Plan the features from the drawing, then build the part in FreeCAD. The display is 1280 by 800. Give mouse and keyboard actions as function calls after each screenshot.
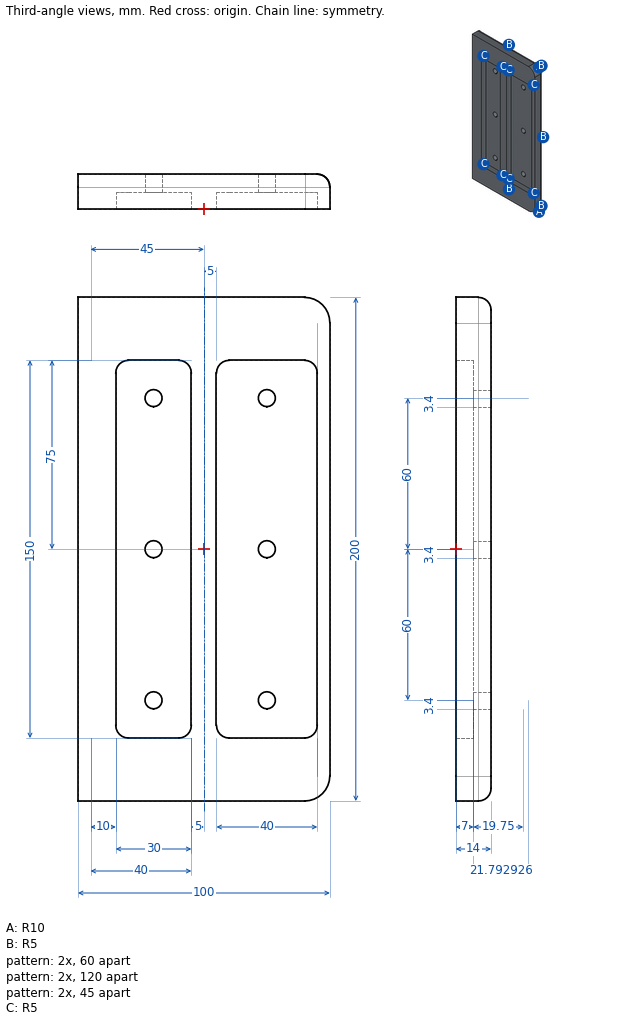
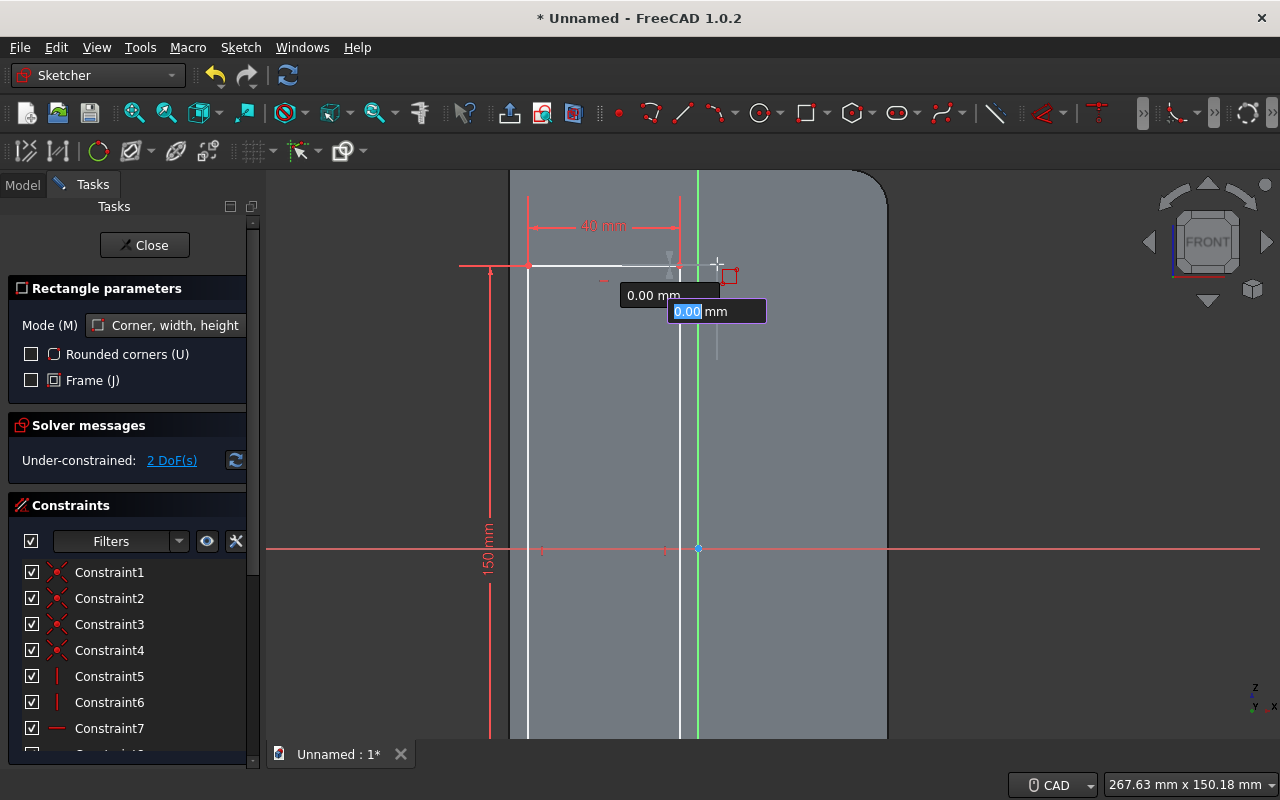
scroll(717, 263, down, 2)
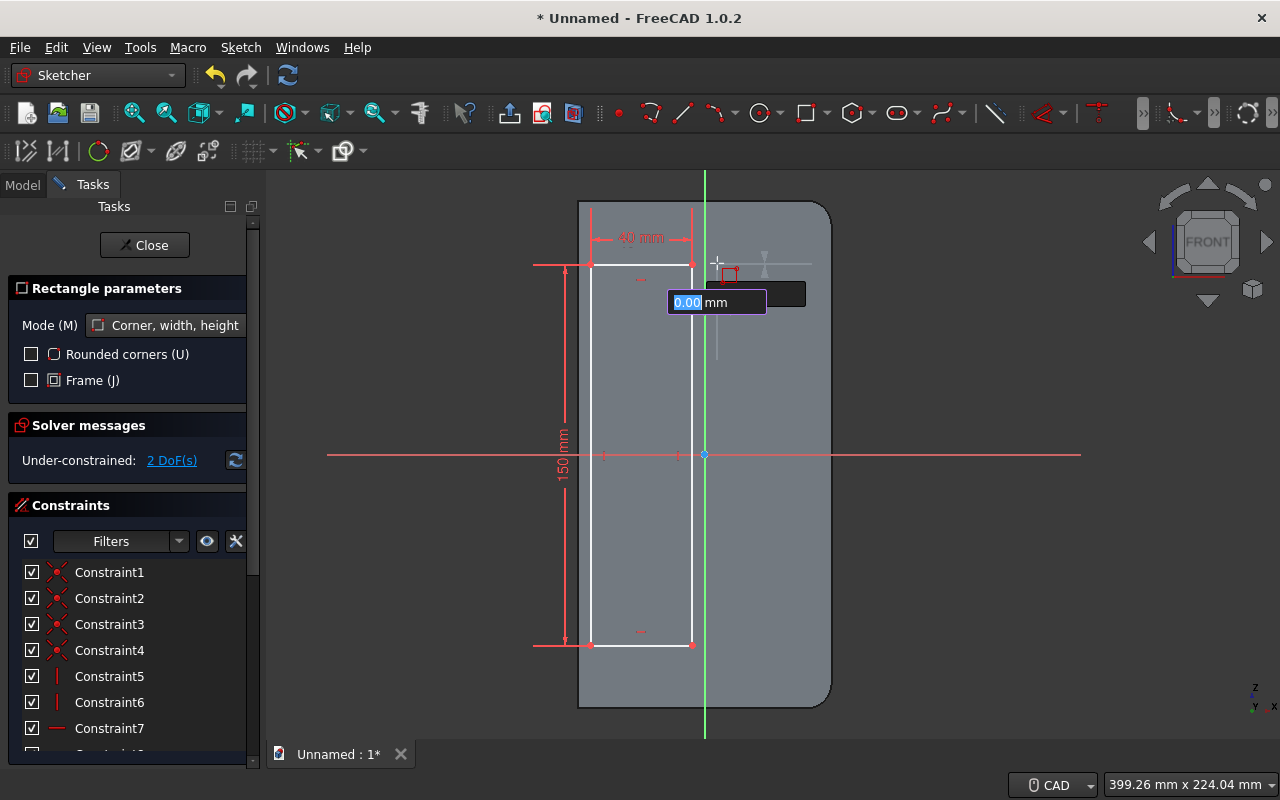
click(819, 645)
key(Escape)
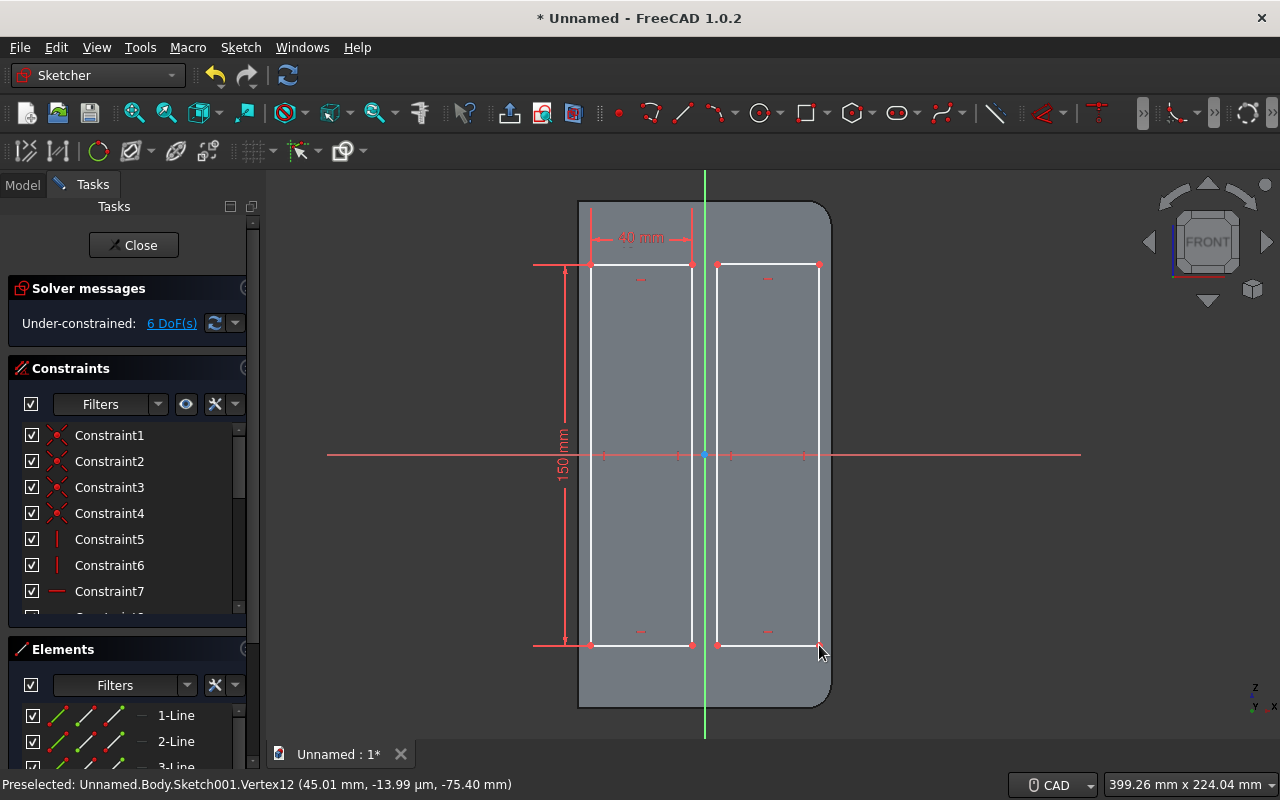
click(692, 265)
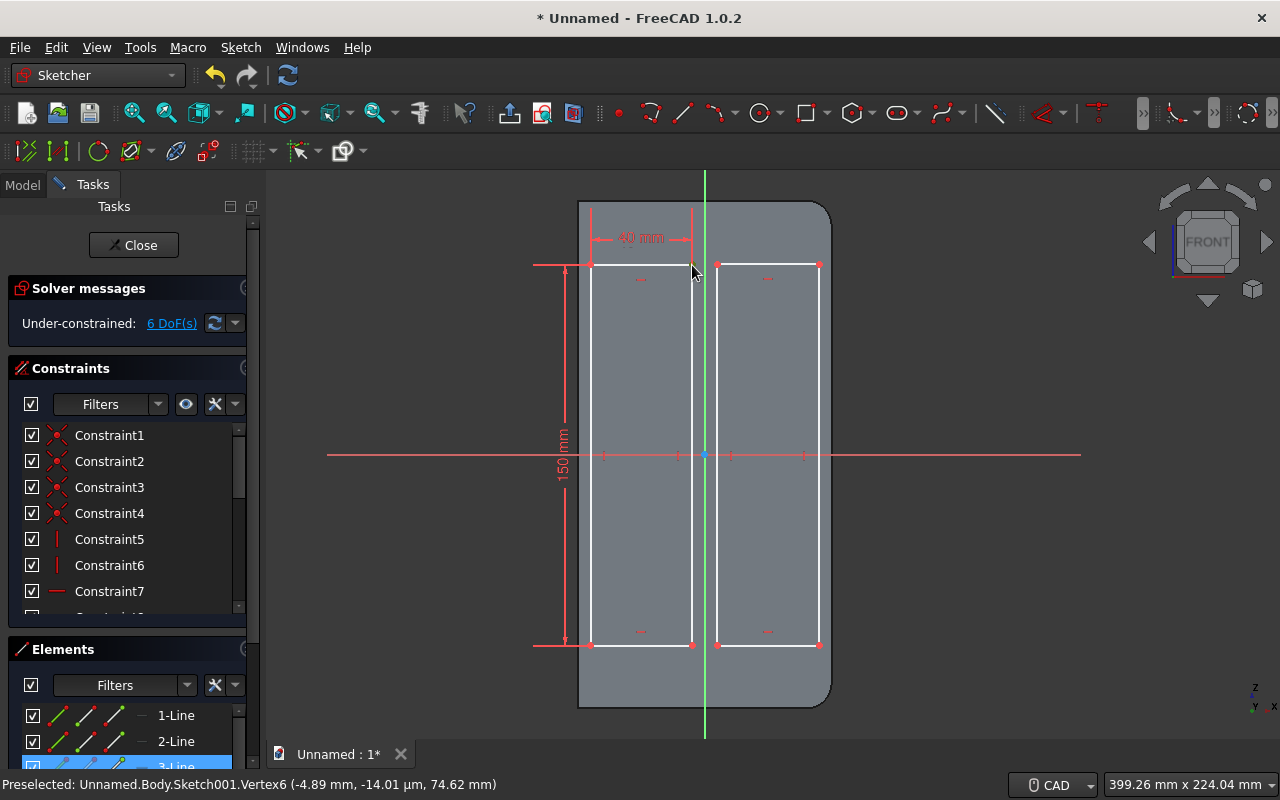
click(717, 264)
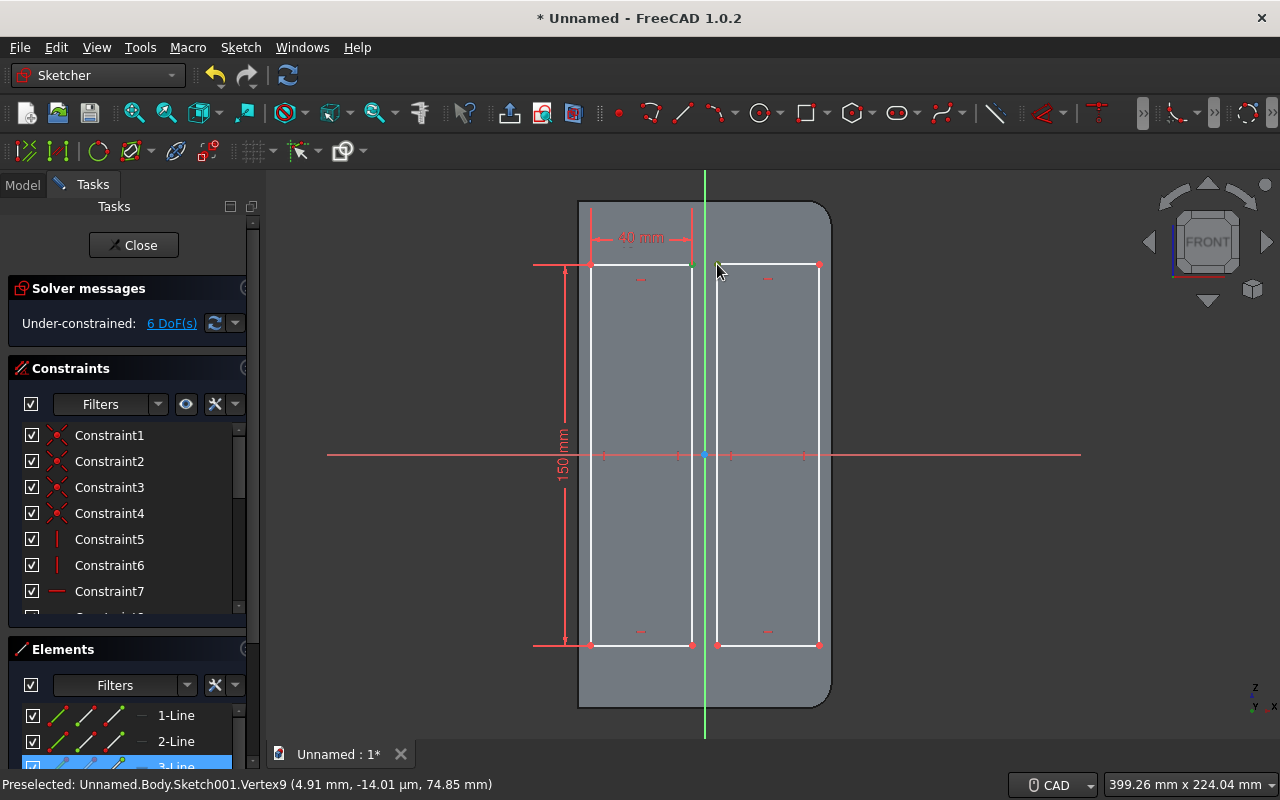
click(705, 674)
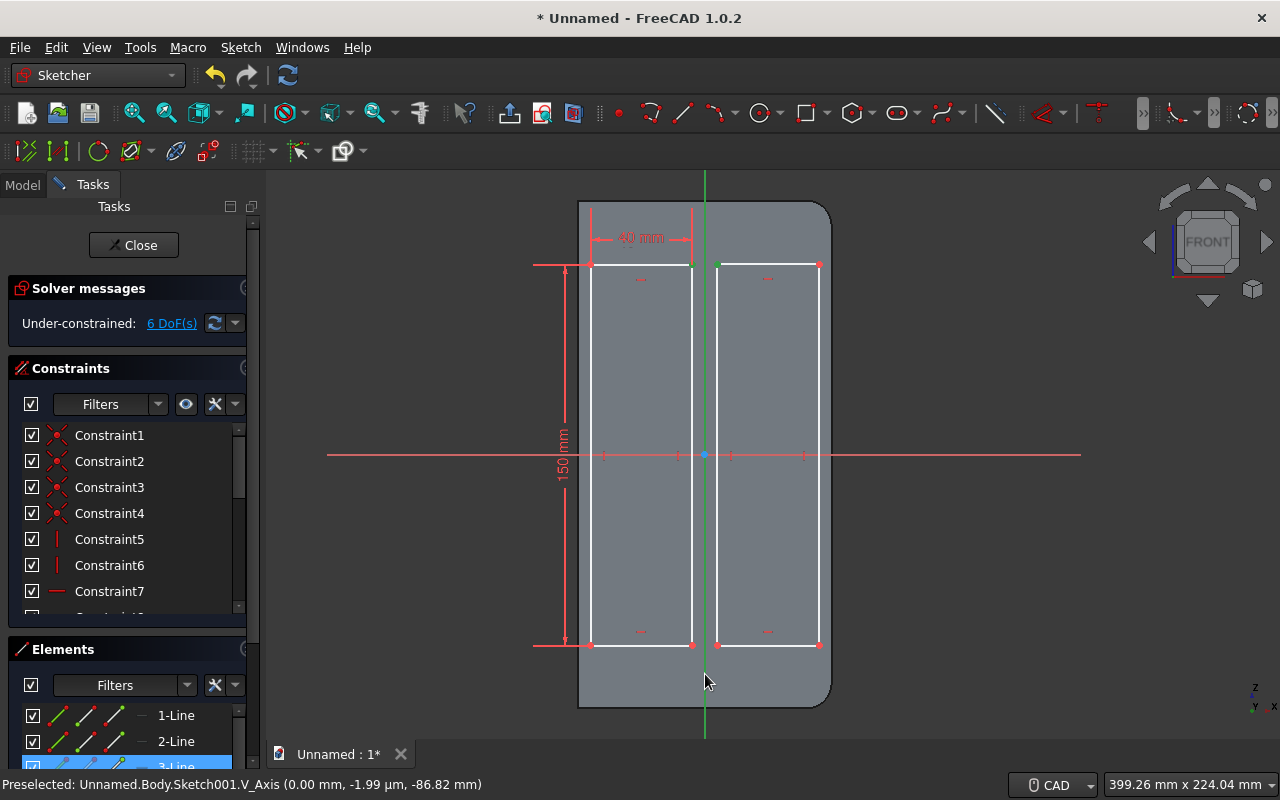
key(s)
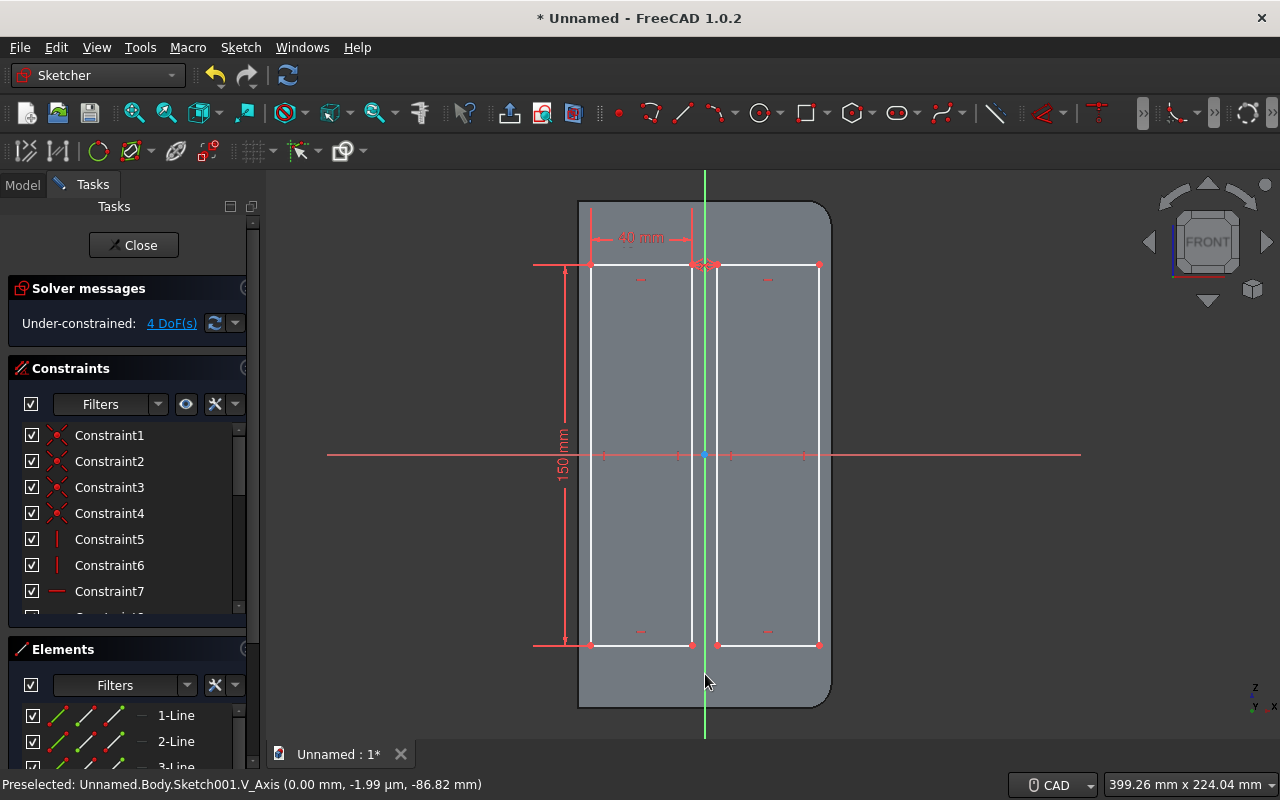
click(591, 646)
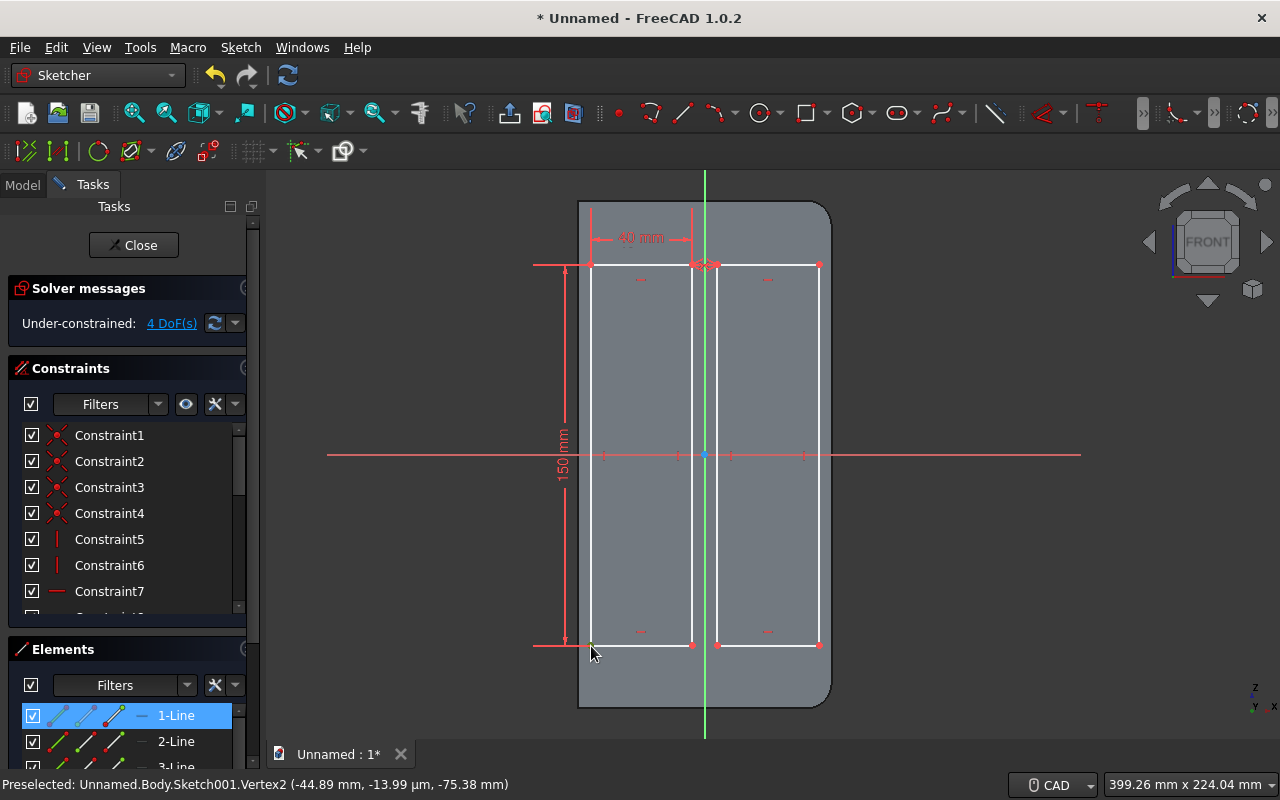
click(819, 646)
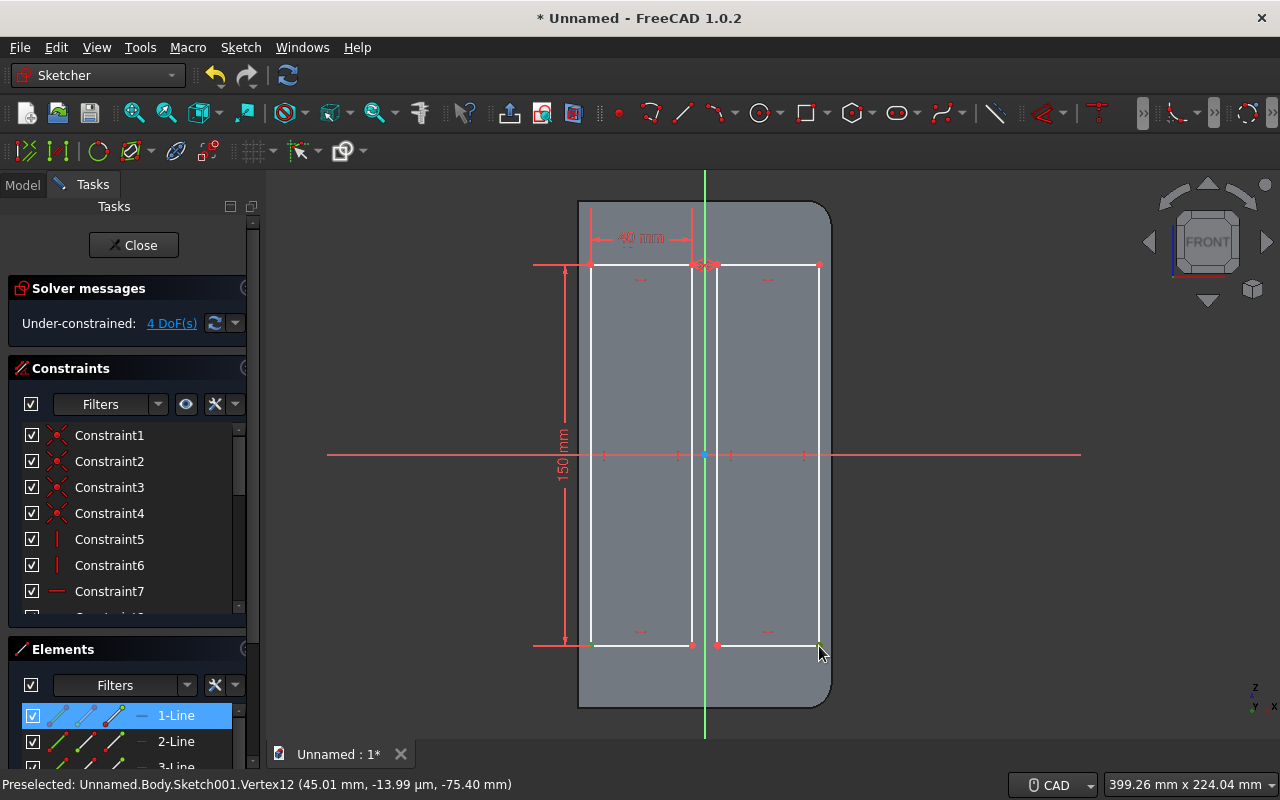
click(705, 674)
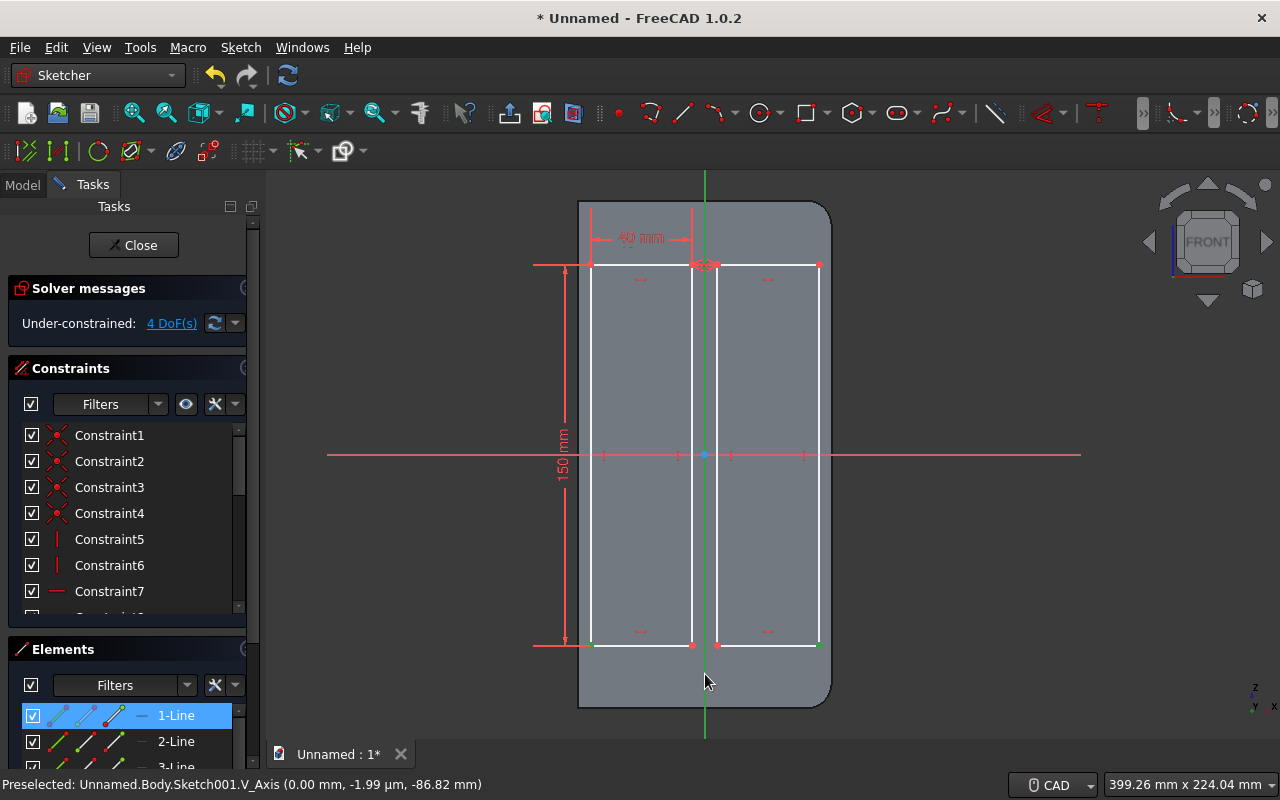
key(s)